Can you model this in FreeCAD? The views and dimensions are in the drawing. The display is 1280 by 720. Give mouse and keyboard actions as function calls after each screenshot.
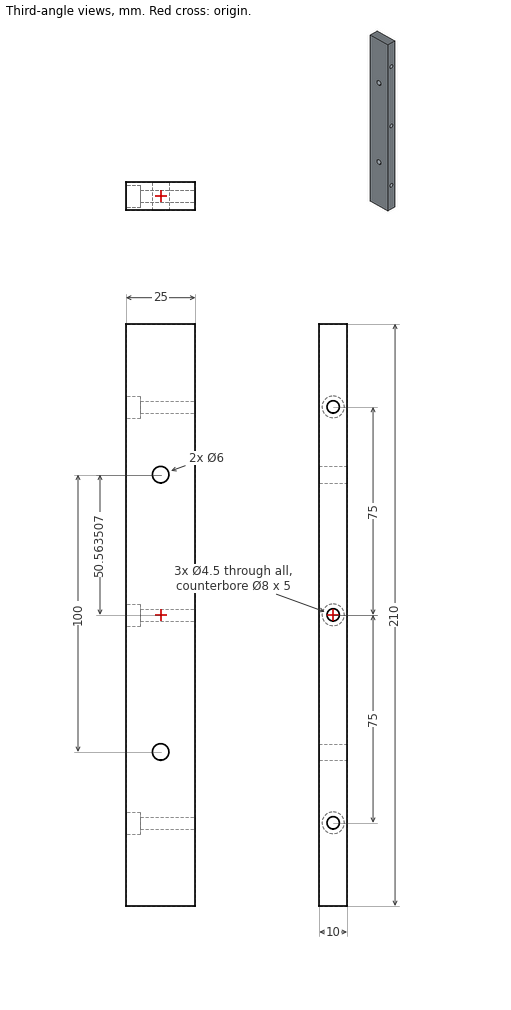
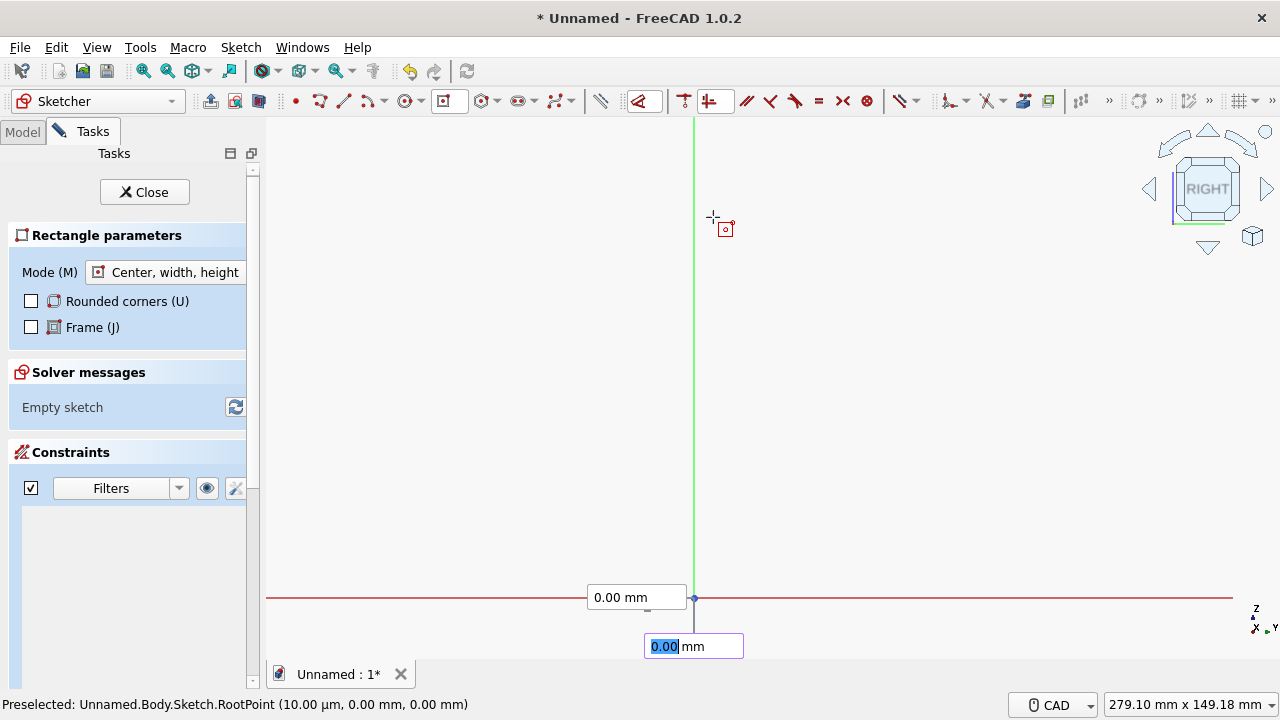
click(712, 217)
key(Escape)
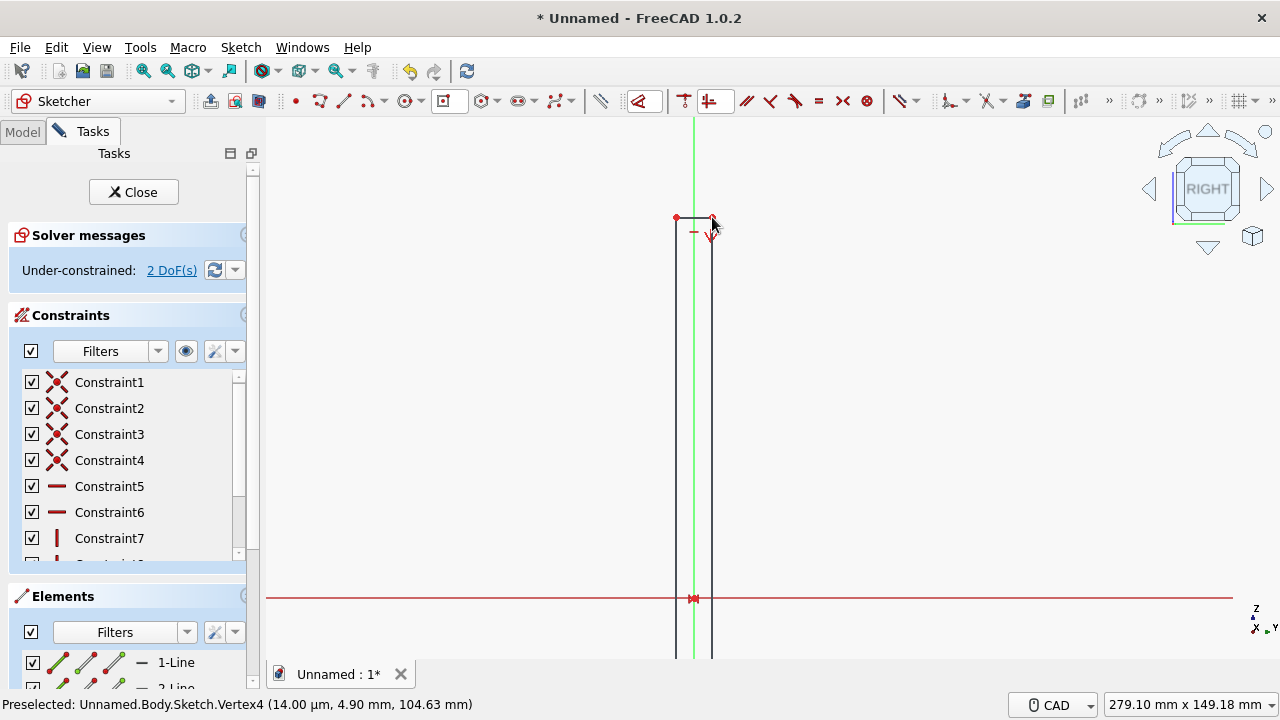
scroll(713, 217, down, 4)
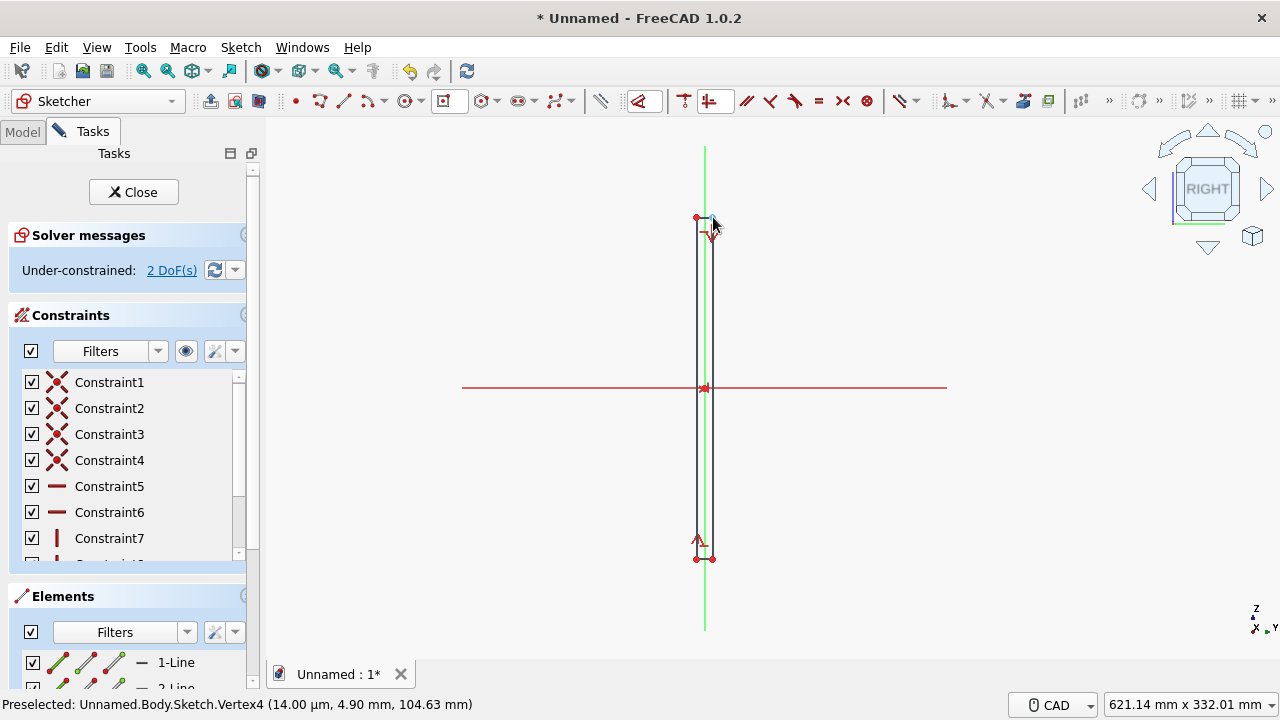
scroll(703, 559, up, 5)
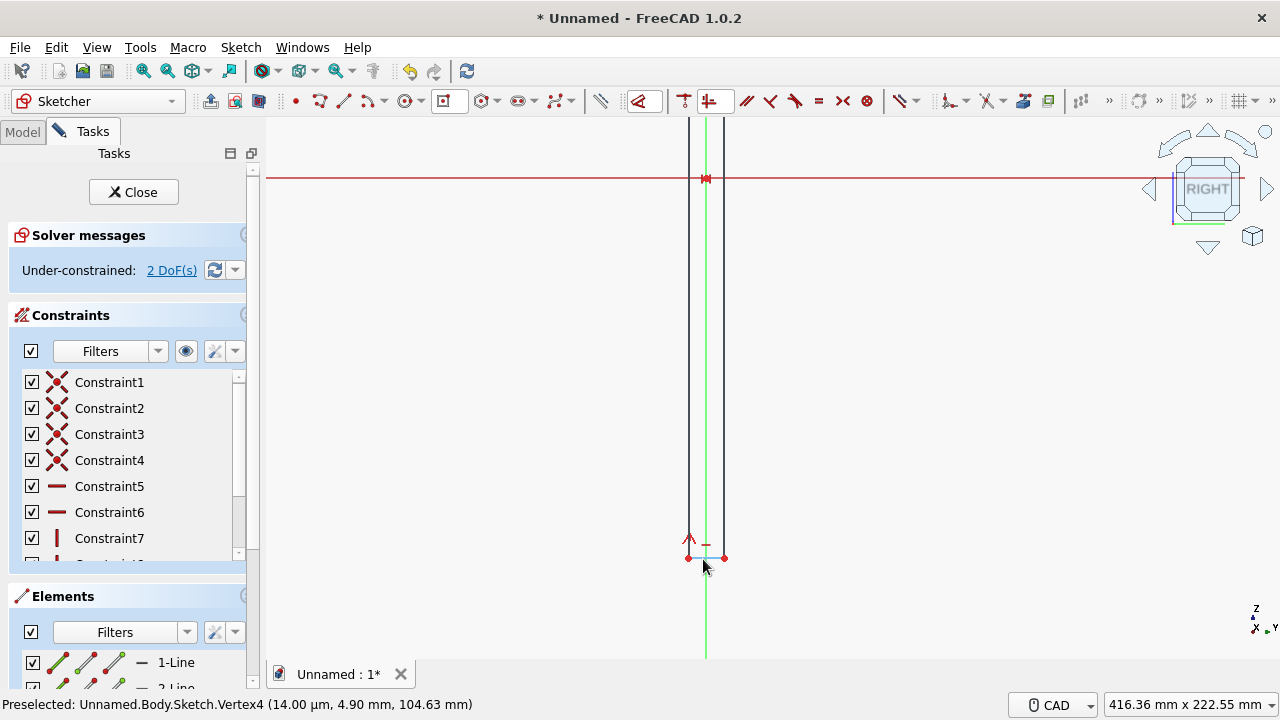
click(703, 558)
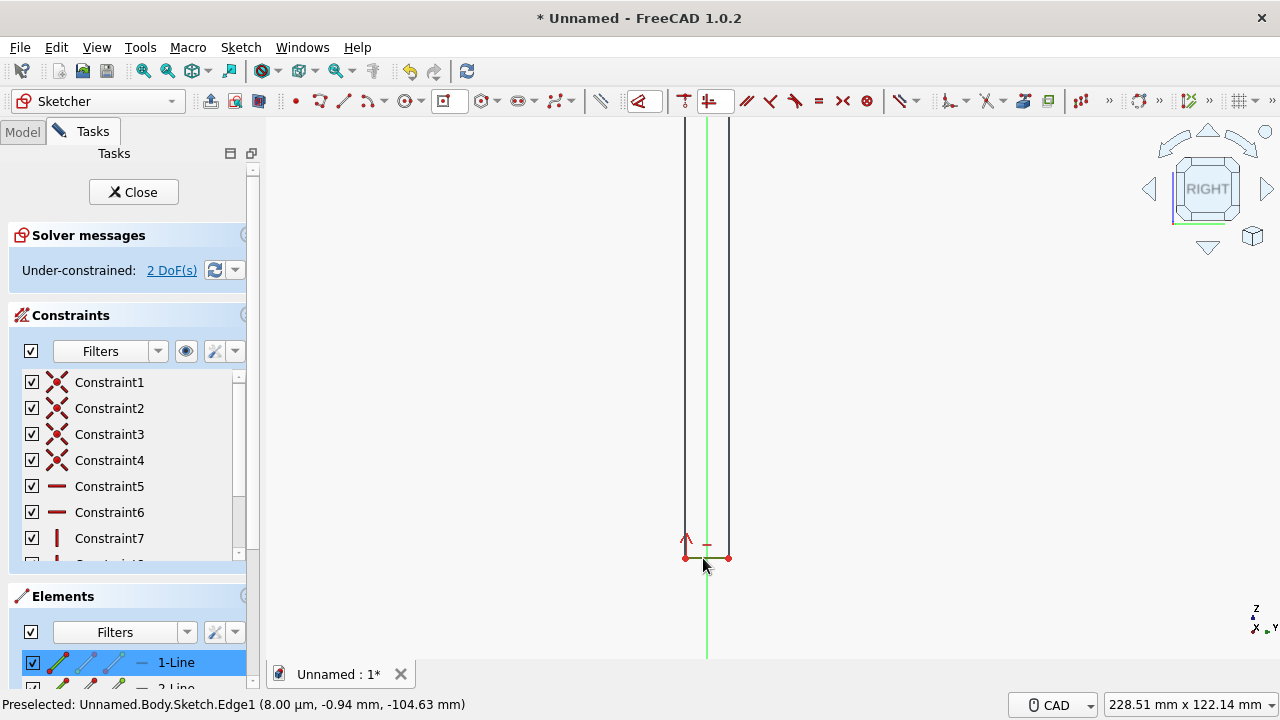
click(656, 102)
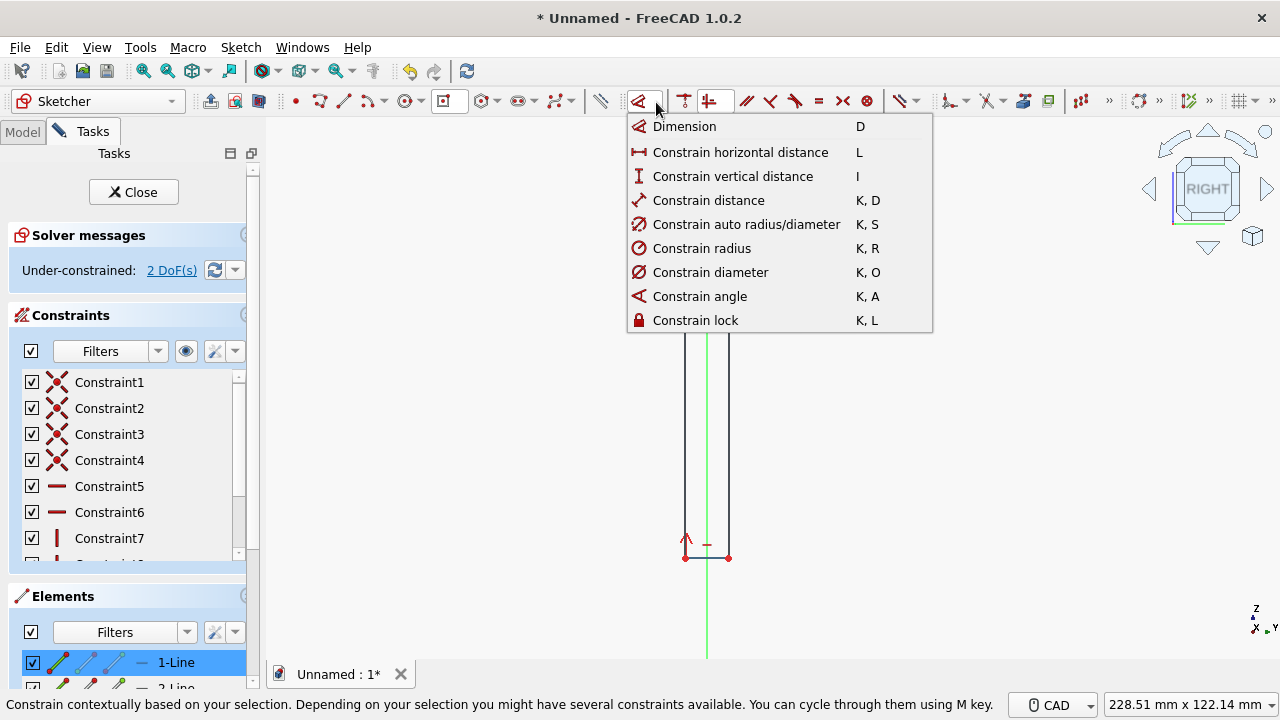
click(780, 152)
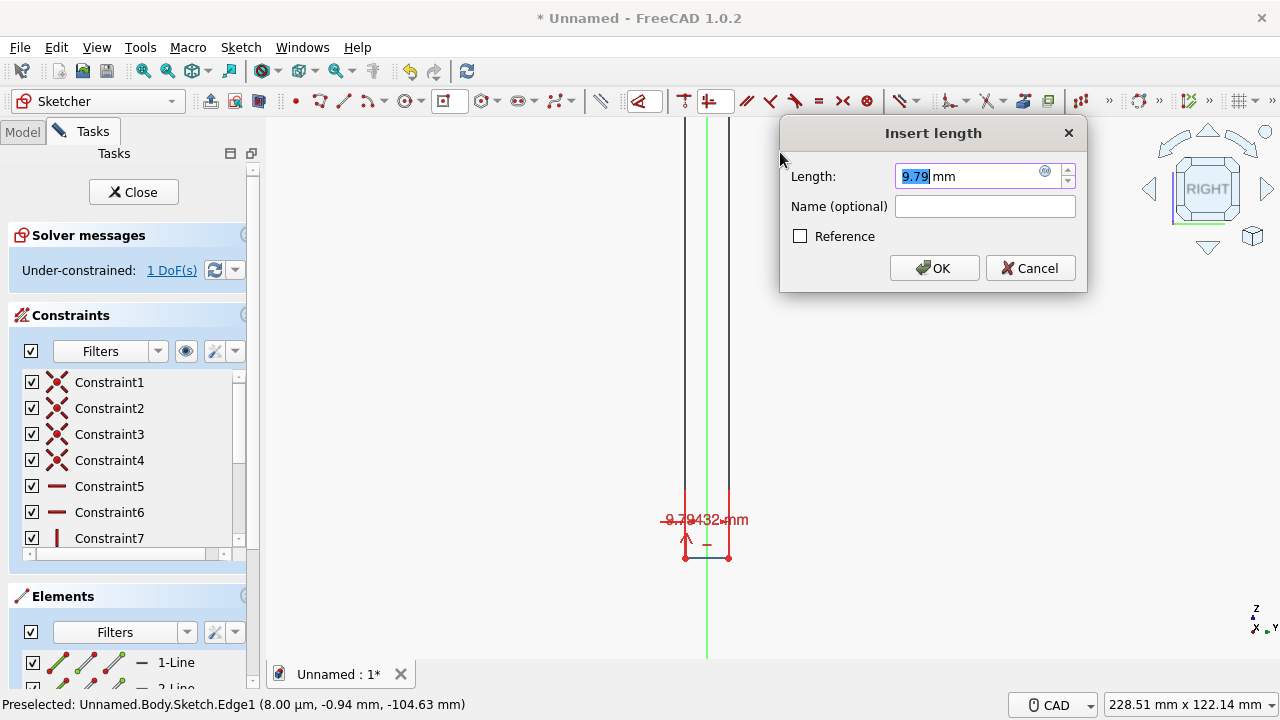
text(10)
key(Return)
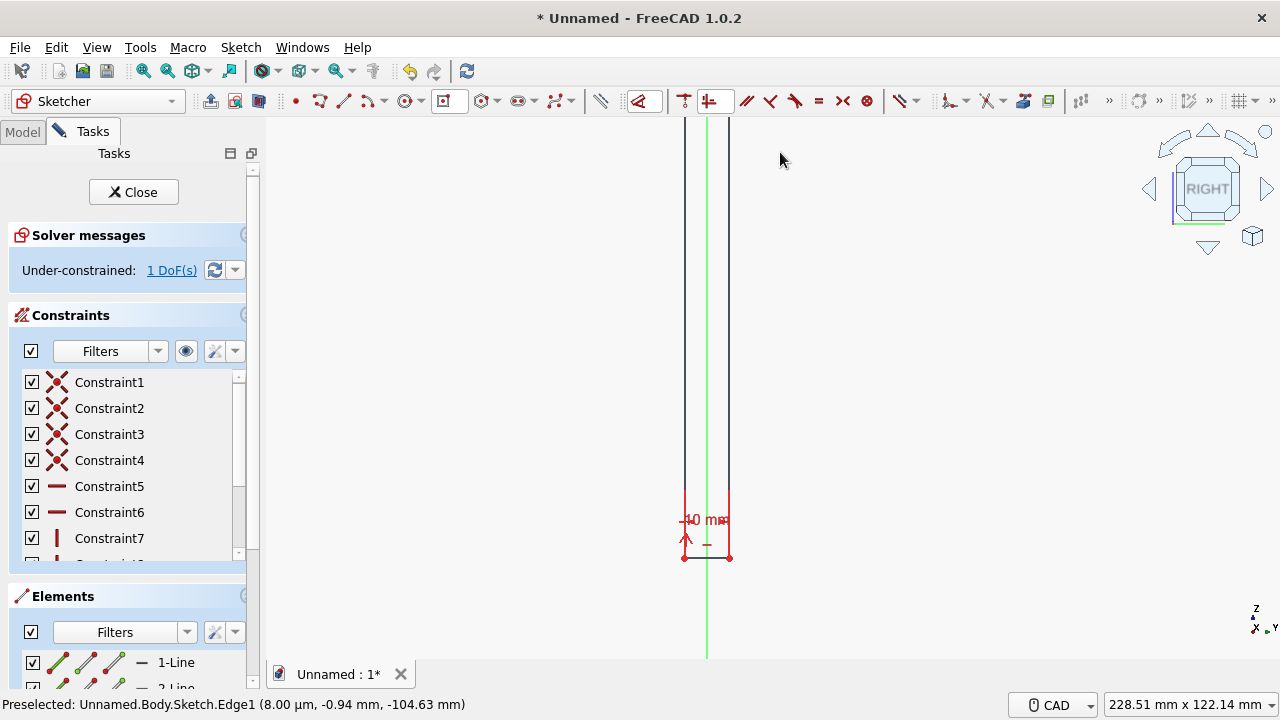
click(729, 279)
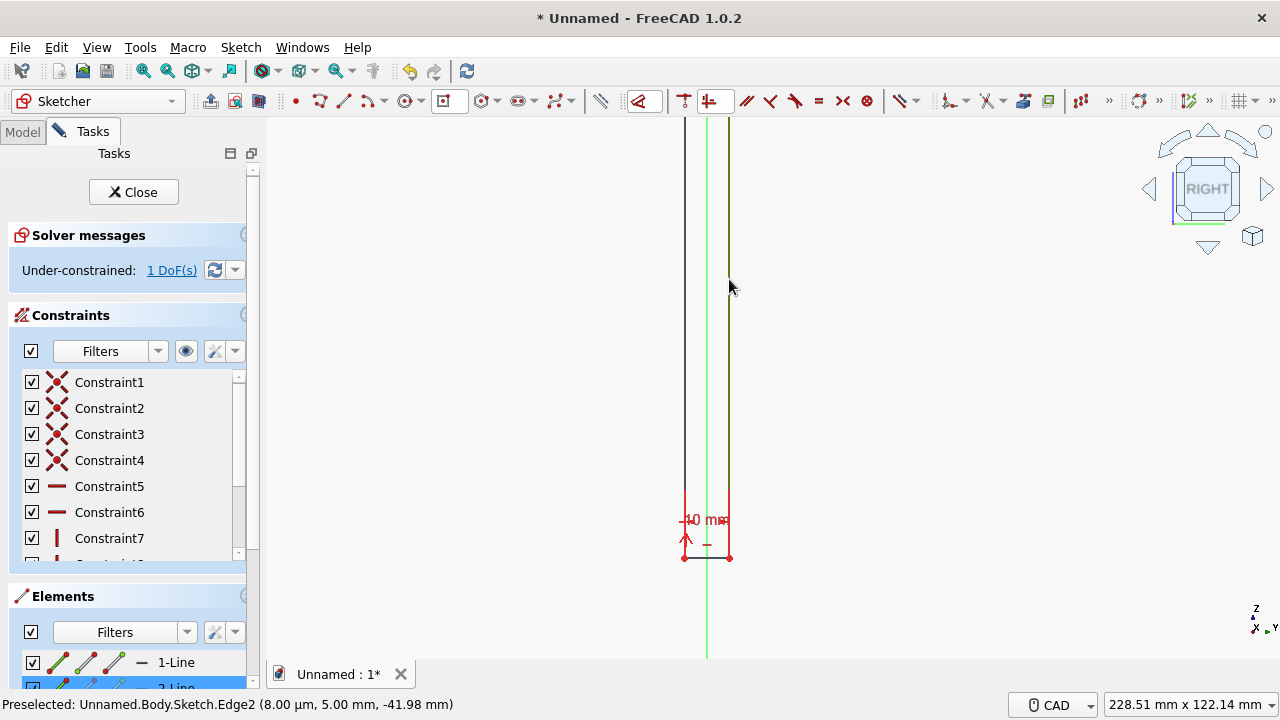
click(656, 102)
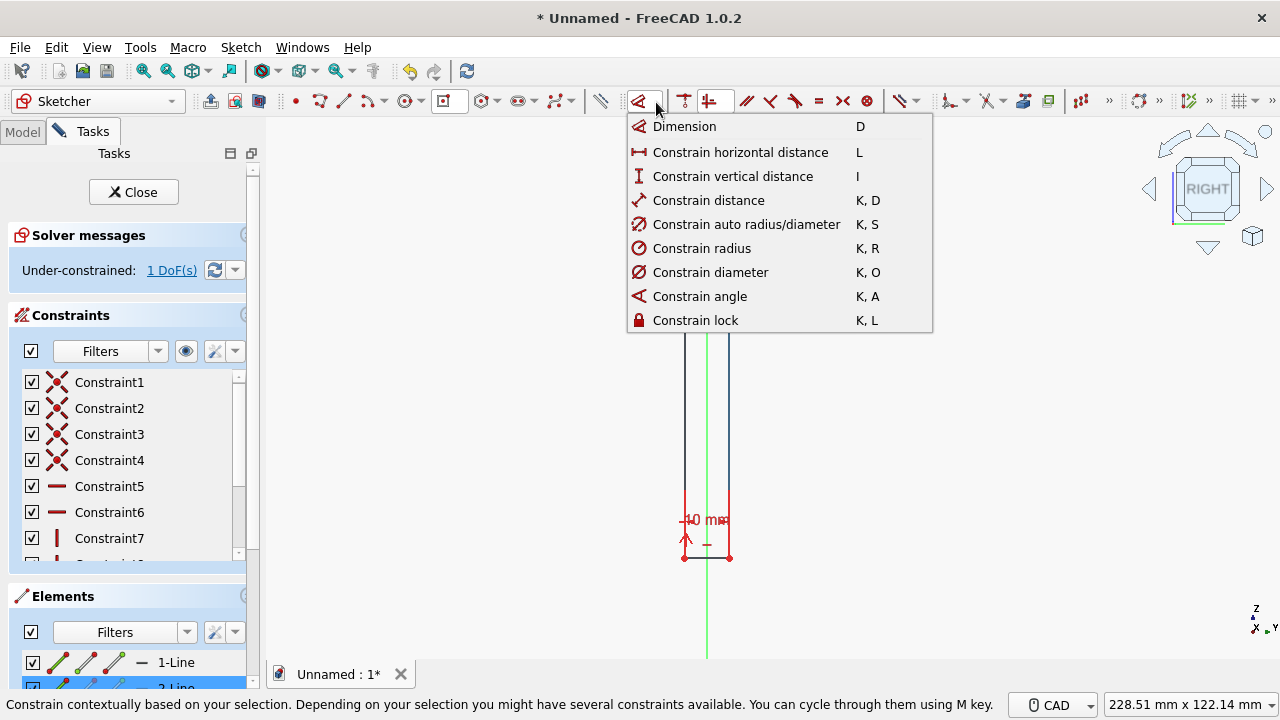
click(780, 176)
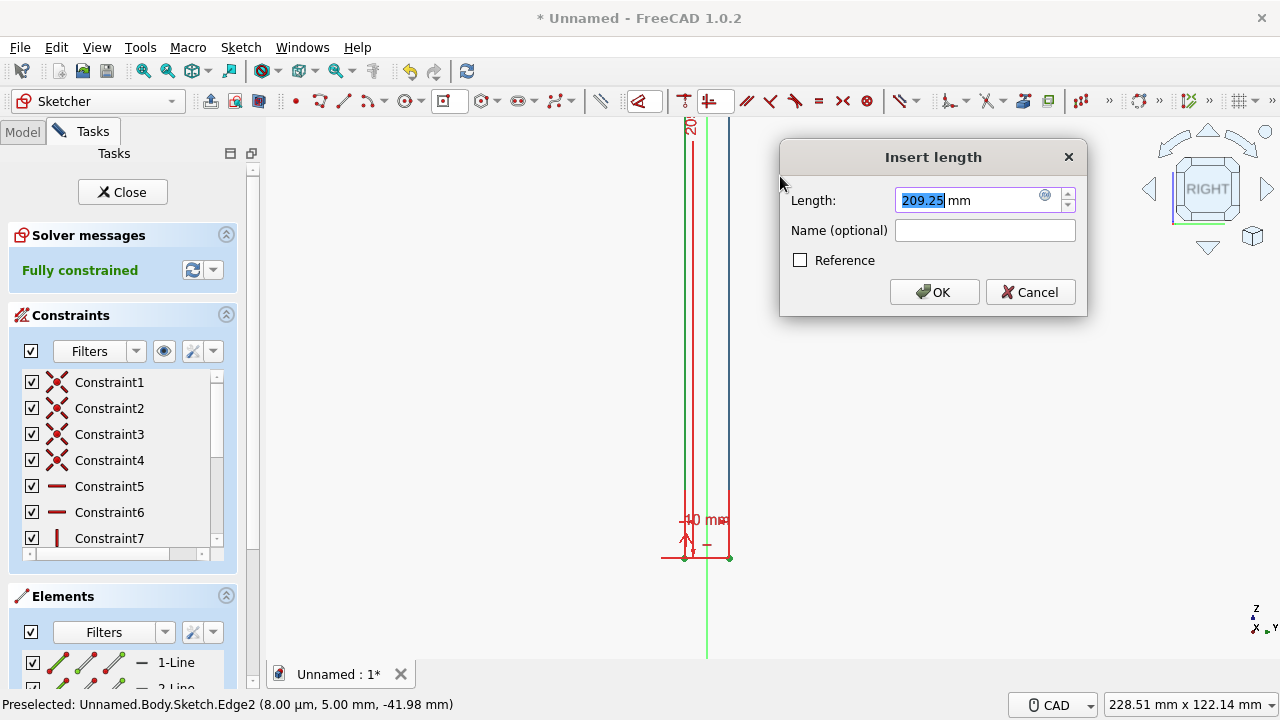
text(210)
key(Return)